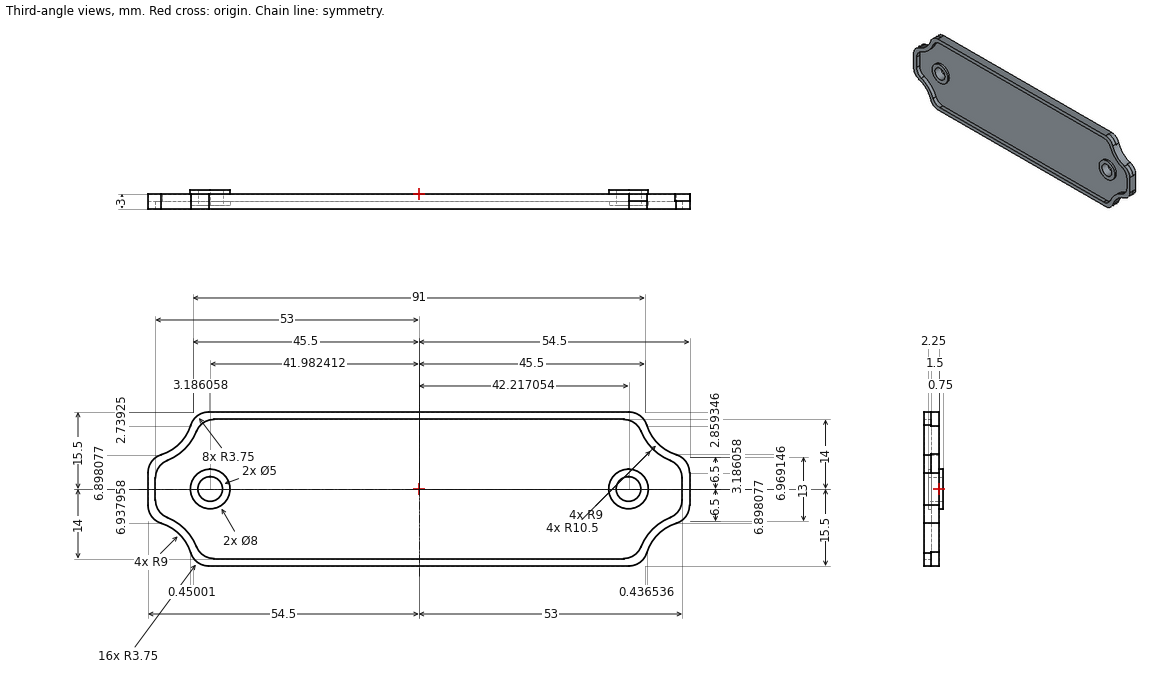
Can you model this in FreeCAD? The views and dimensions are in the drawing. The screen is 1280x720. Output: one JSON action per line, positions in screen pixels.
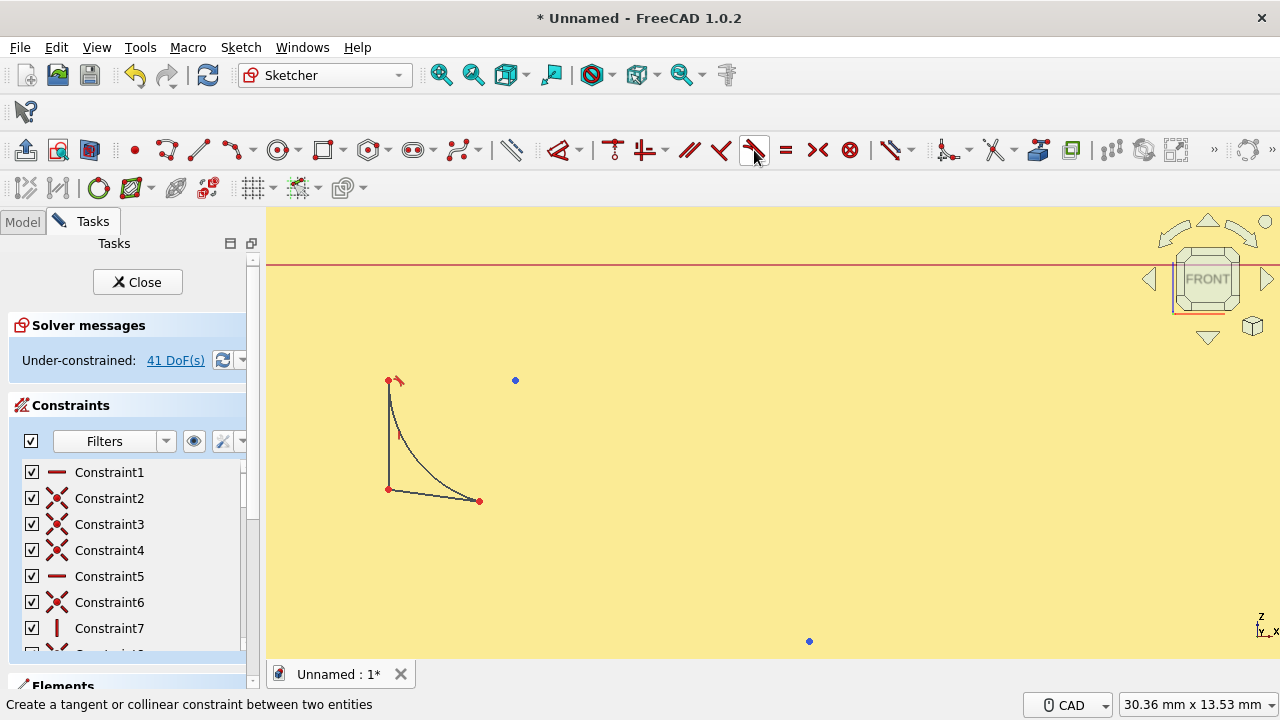
{"action": "scroll", "coordinate": [407, 466], "scroll_direction": "down", "scroll_amount": 9}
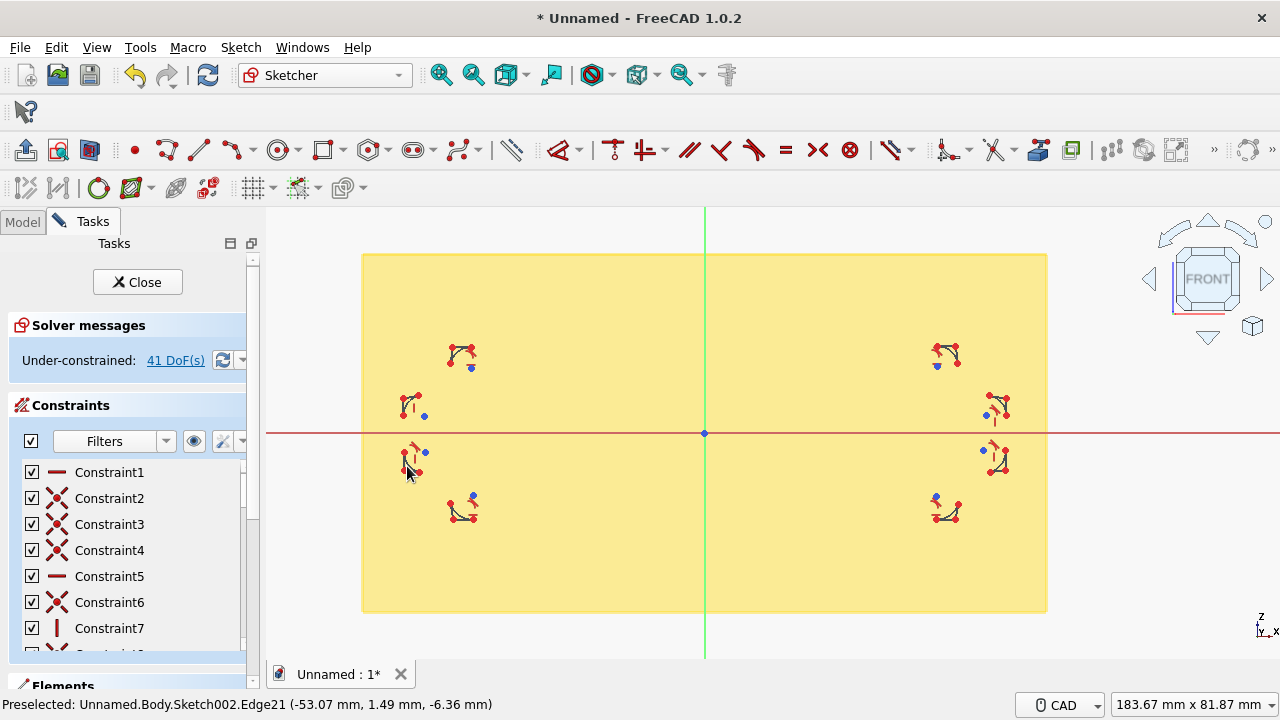
{"action": "scroll", "coordinate": [403, 404], "scroll_direction": "up", "scroll_amount": 8}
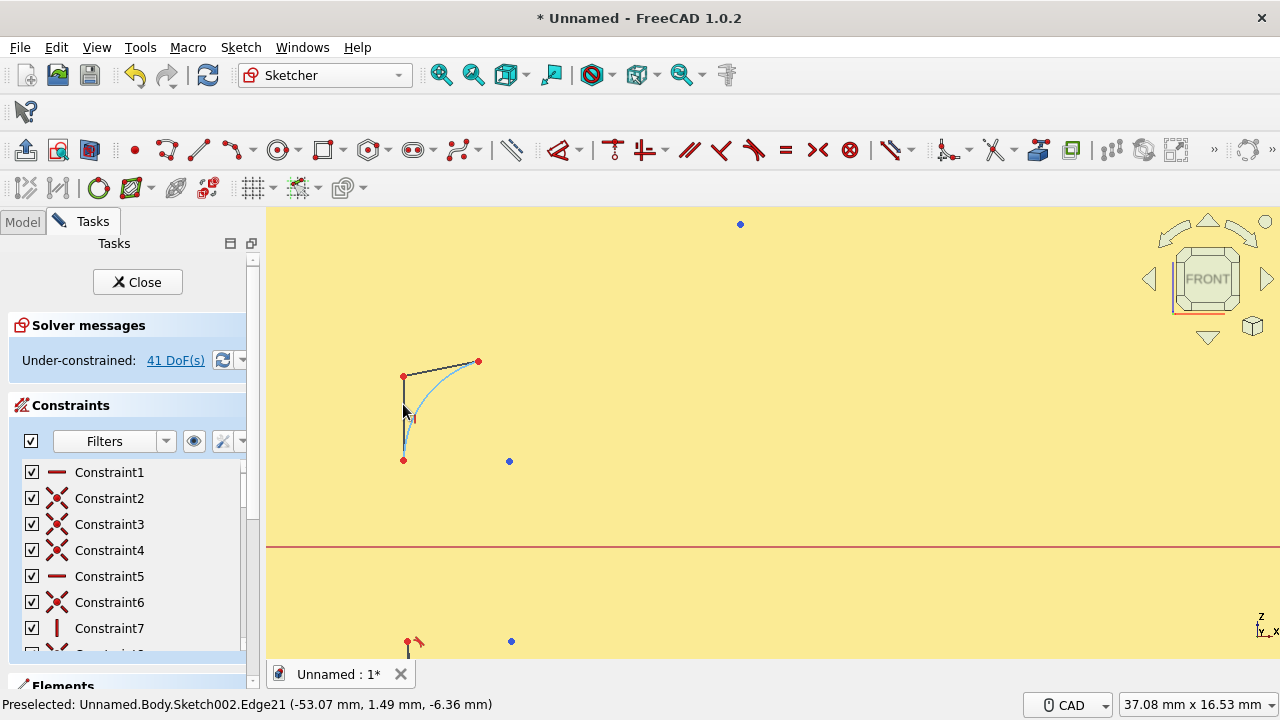
{"action": "left_click", "coordinate": [404, 401]}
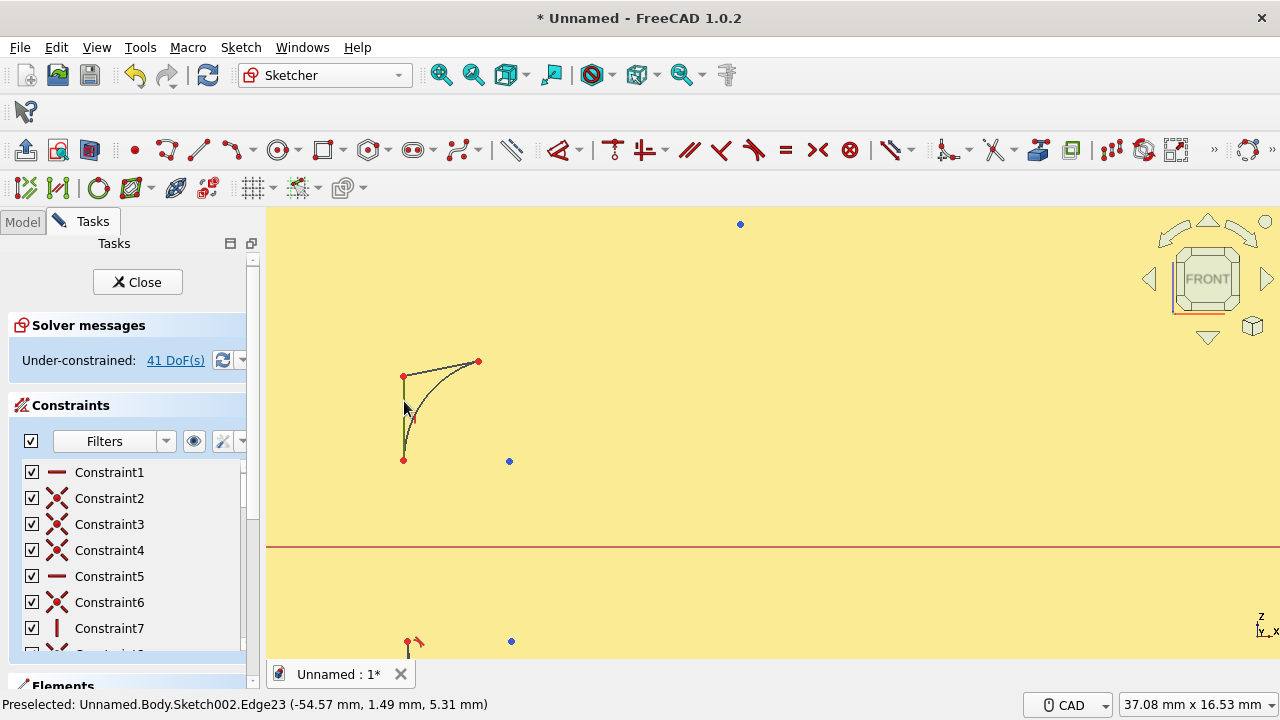
{"action": "left_click", "coordinate": [443, 380]}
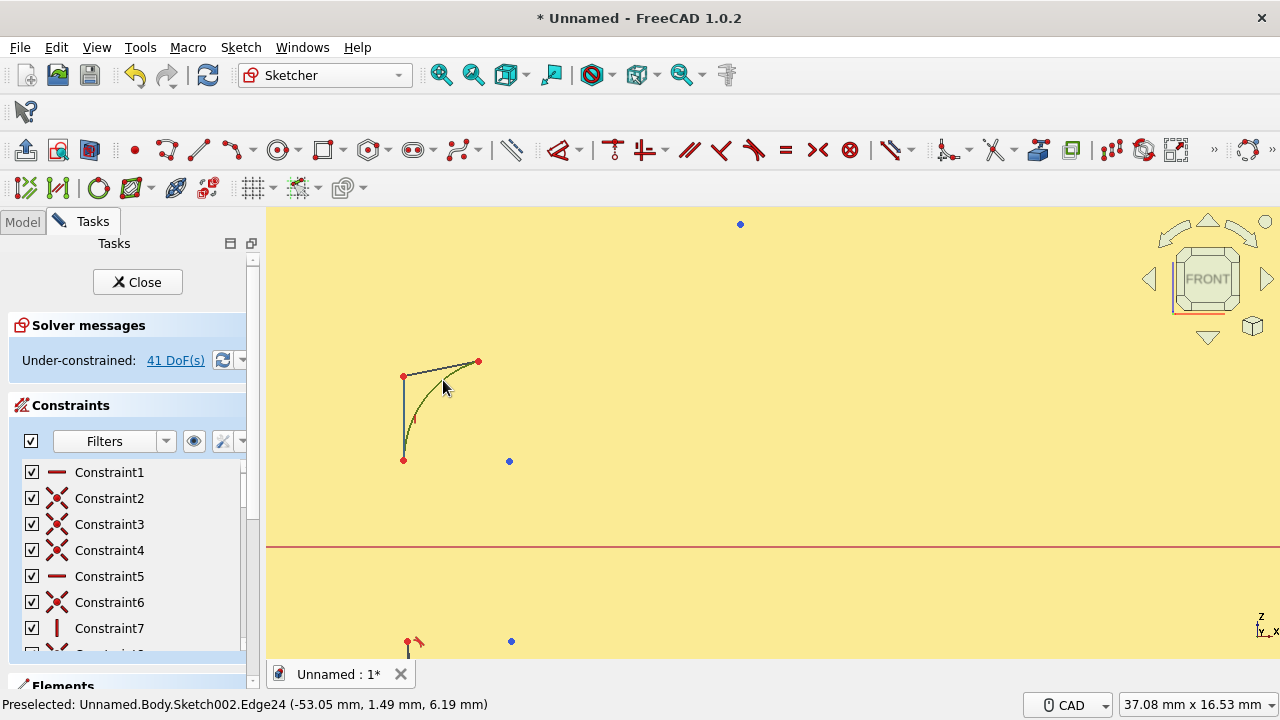
{"action": "left_click", "coordinate": [754, 150]}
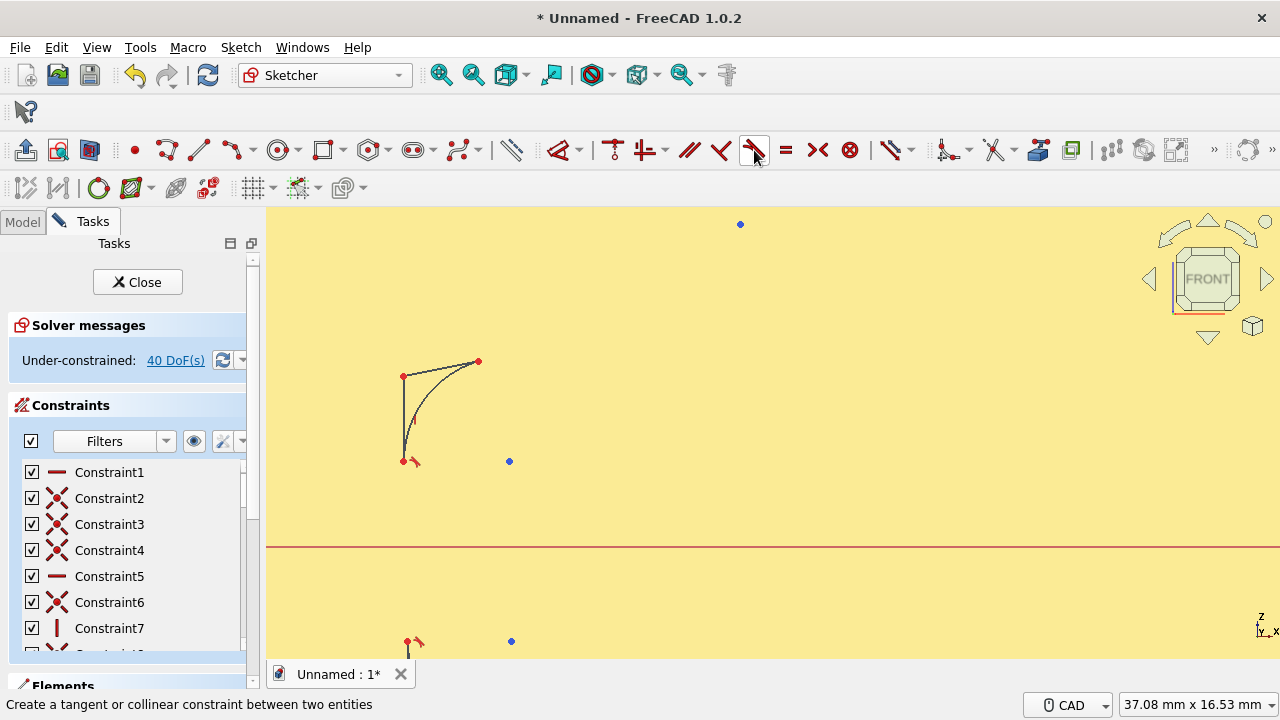
{"action": "scroll", "coordinate": [403, 404], "scroll_direction": "down", "scroll_amount": 8}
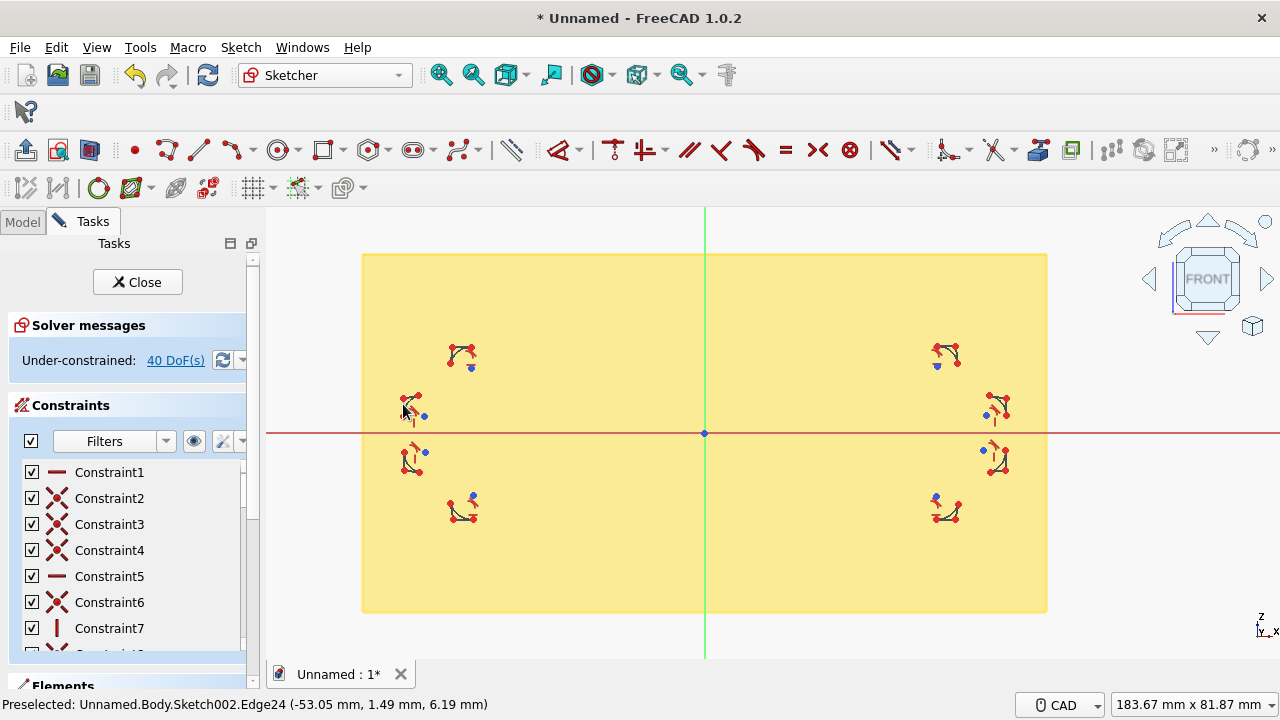
{"action": "scroll", "coordinate": [454, 356], "scroll_direction": "up", "scroll_amount": 9}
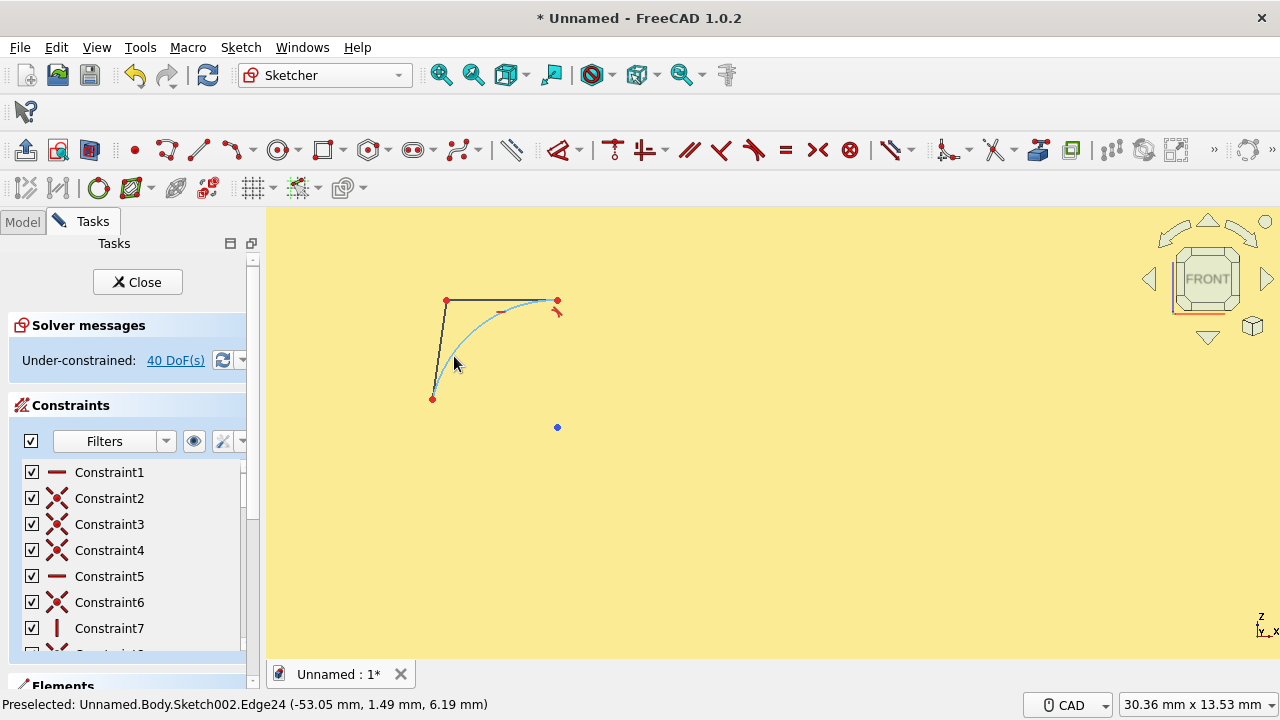
{"action": "left_click", "coordinate": [454, 353]}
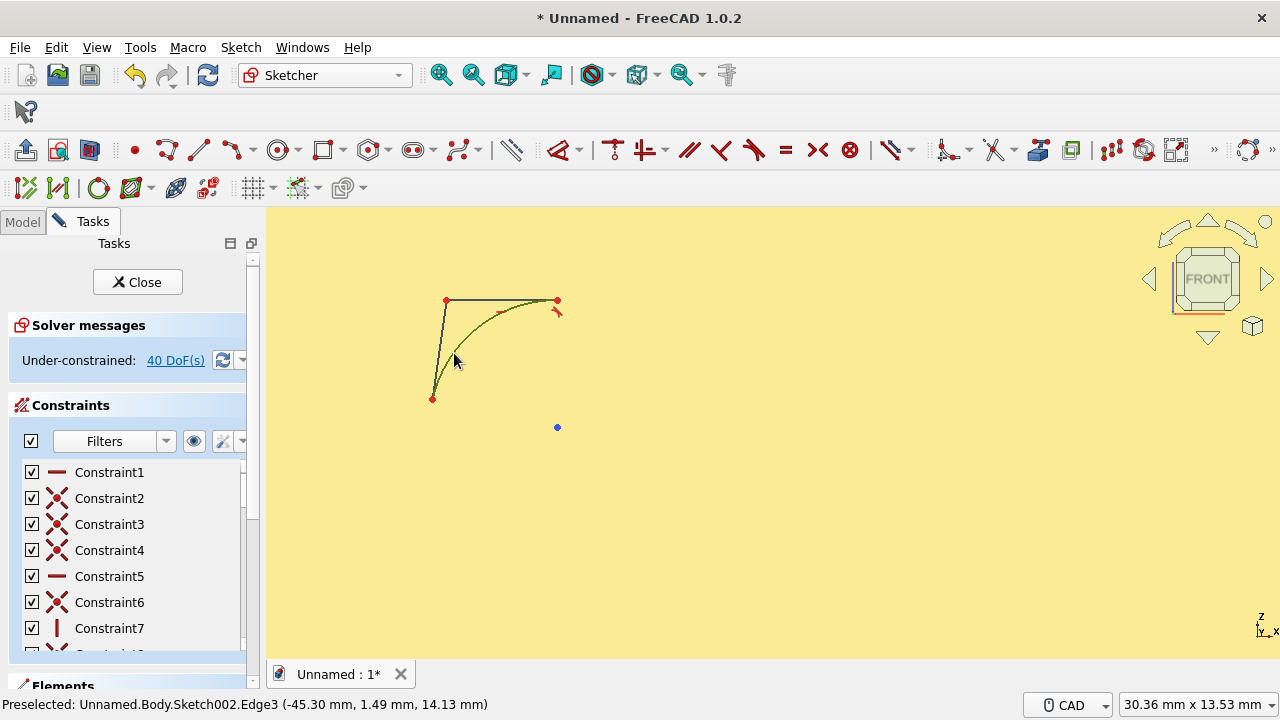
{"action": "scroll", "coordinate": [454, 356], "scroll_direction": "down", "scroll_amount": 9}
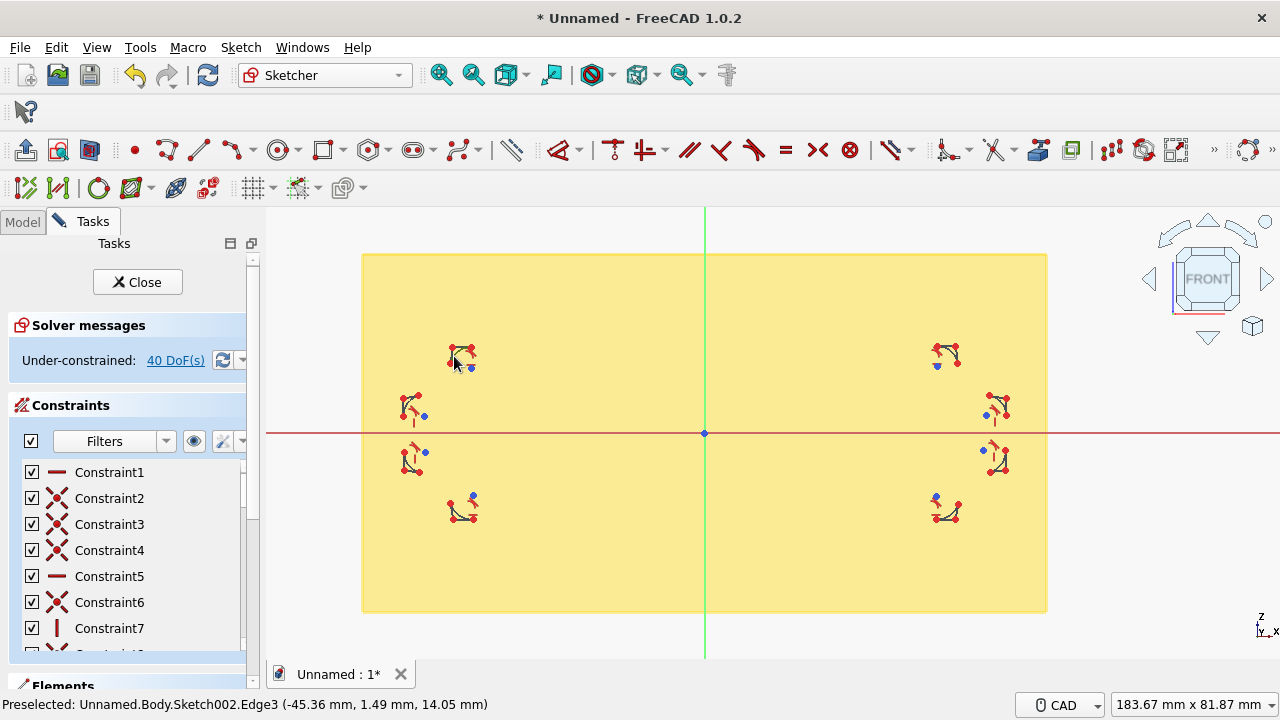
{"action": "scroll", "coordinate": [955, 356], "scroll_direction": "up", "scroll_amount": 10}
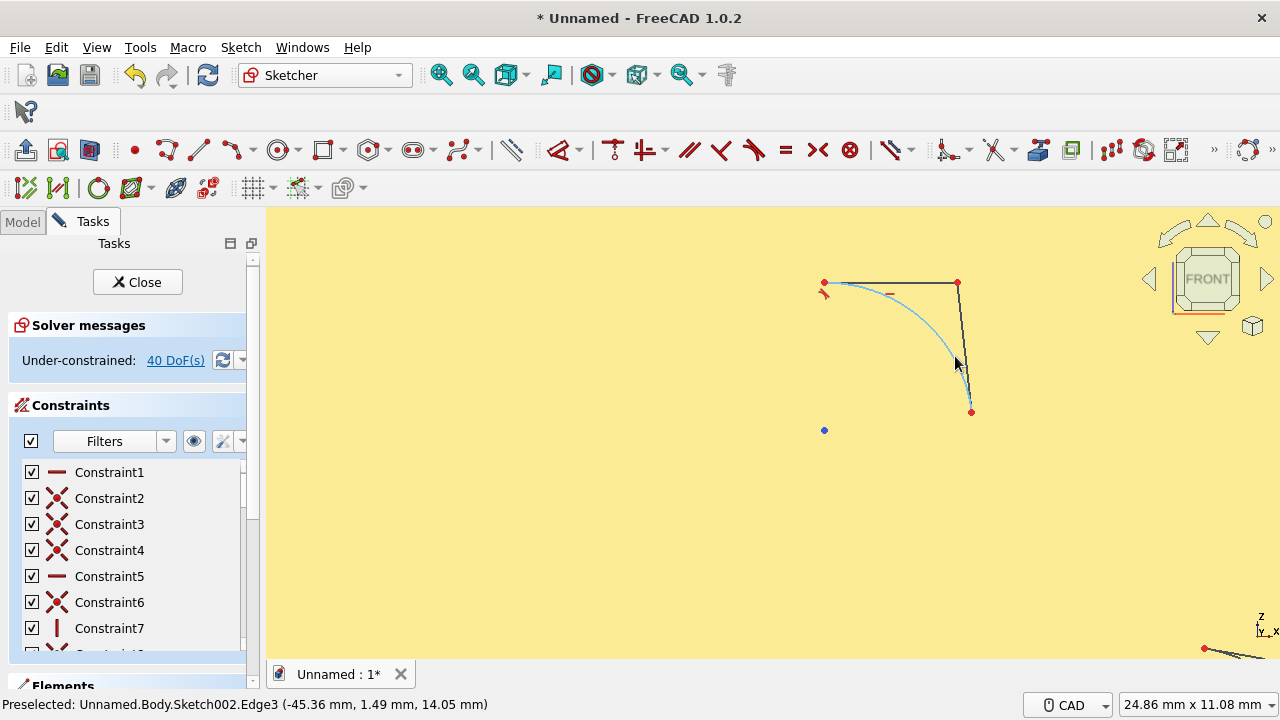
{"action": "left_click", "coordinate": [951, 353]}